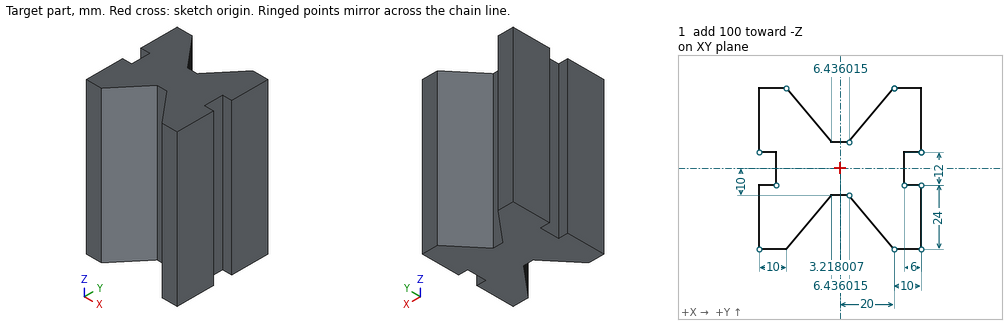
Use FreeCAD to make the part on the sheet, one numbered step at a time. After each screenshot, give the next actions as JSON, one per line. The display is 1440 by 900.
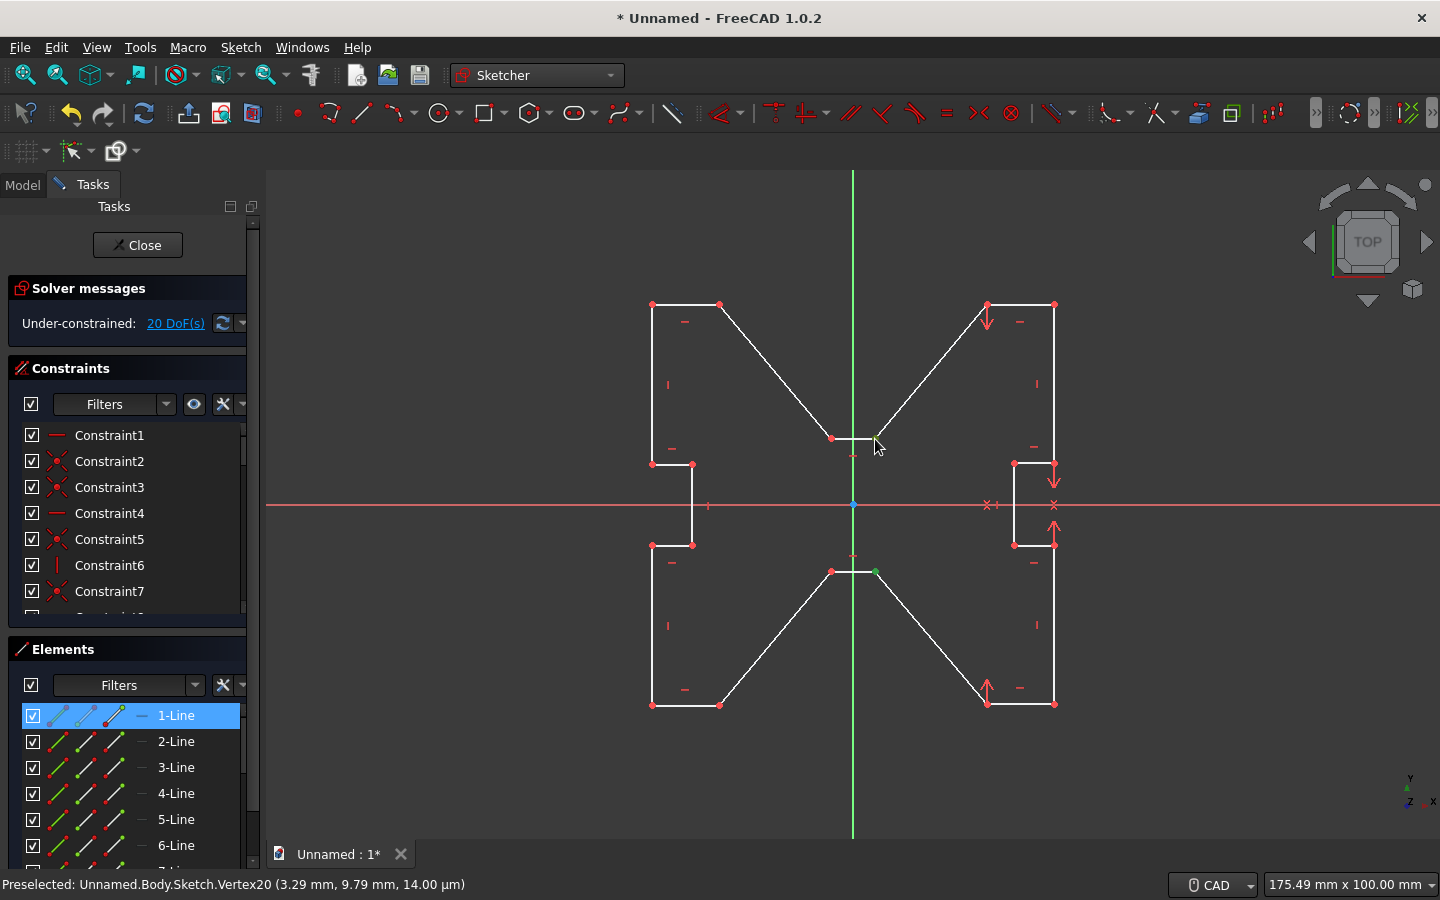
{"action": "left_click", "coordinate": [364, 504]}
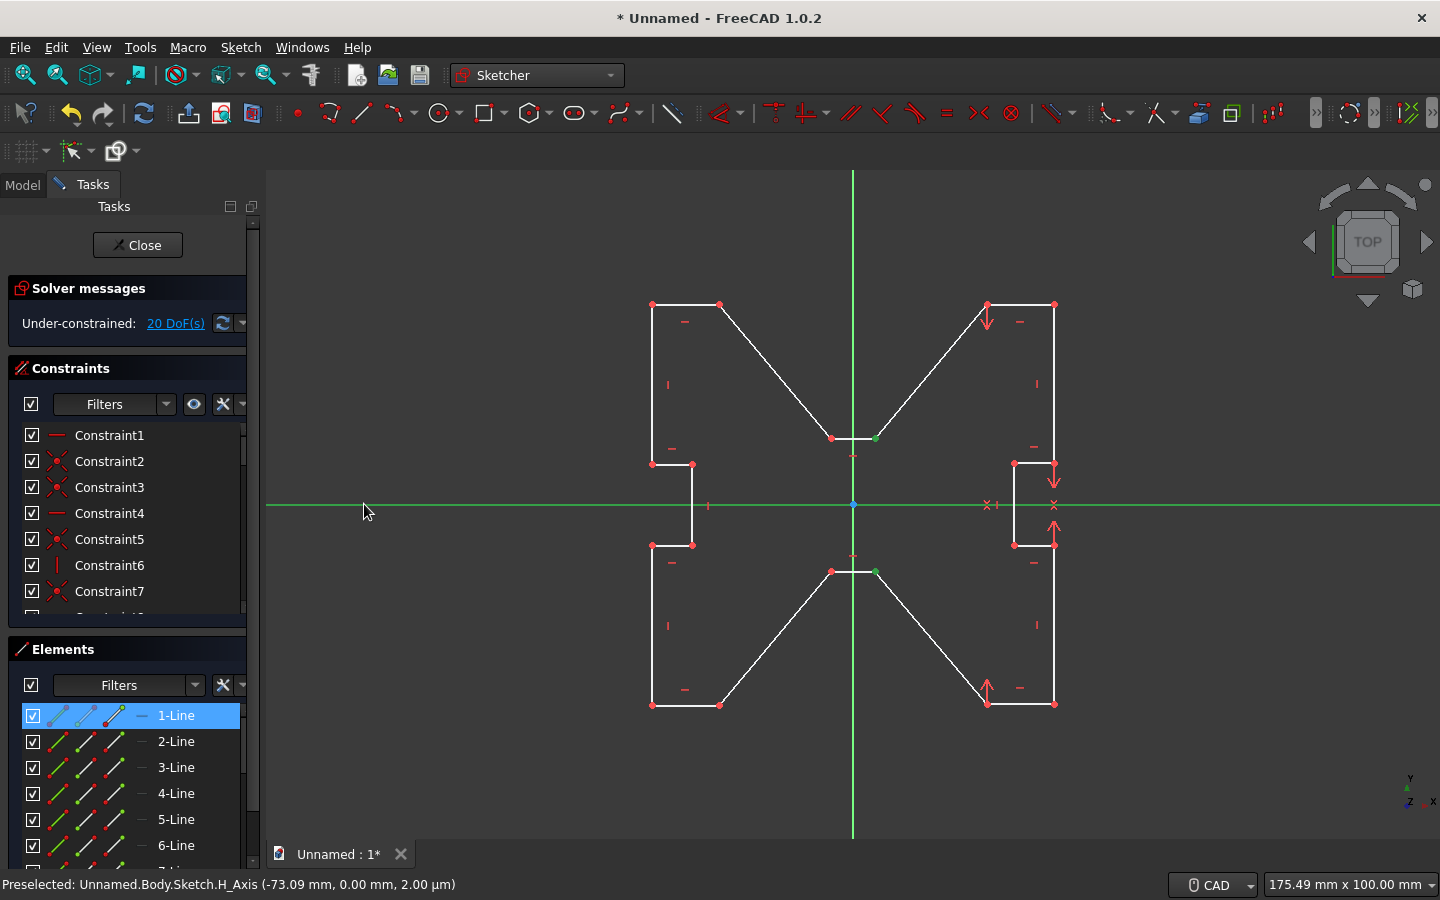
{"action": "key", "text": "s"}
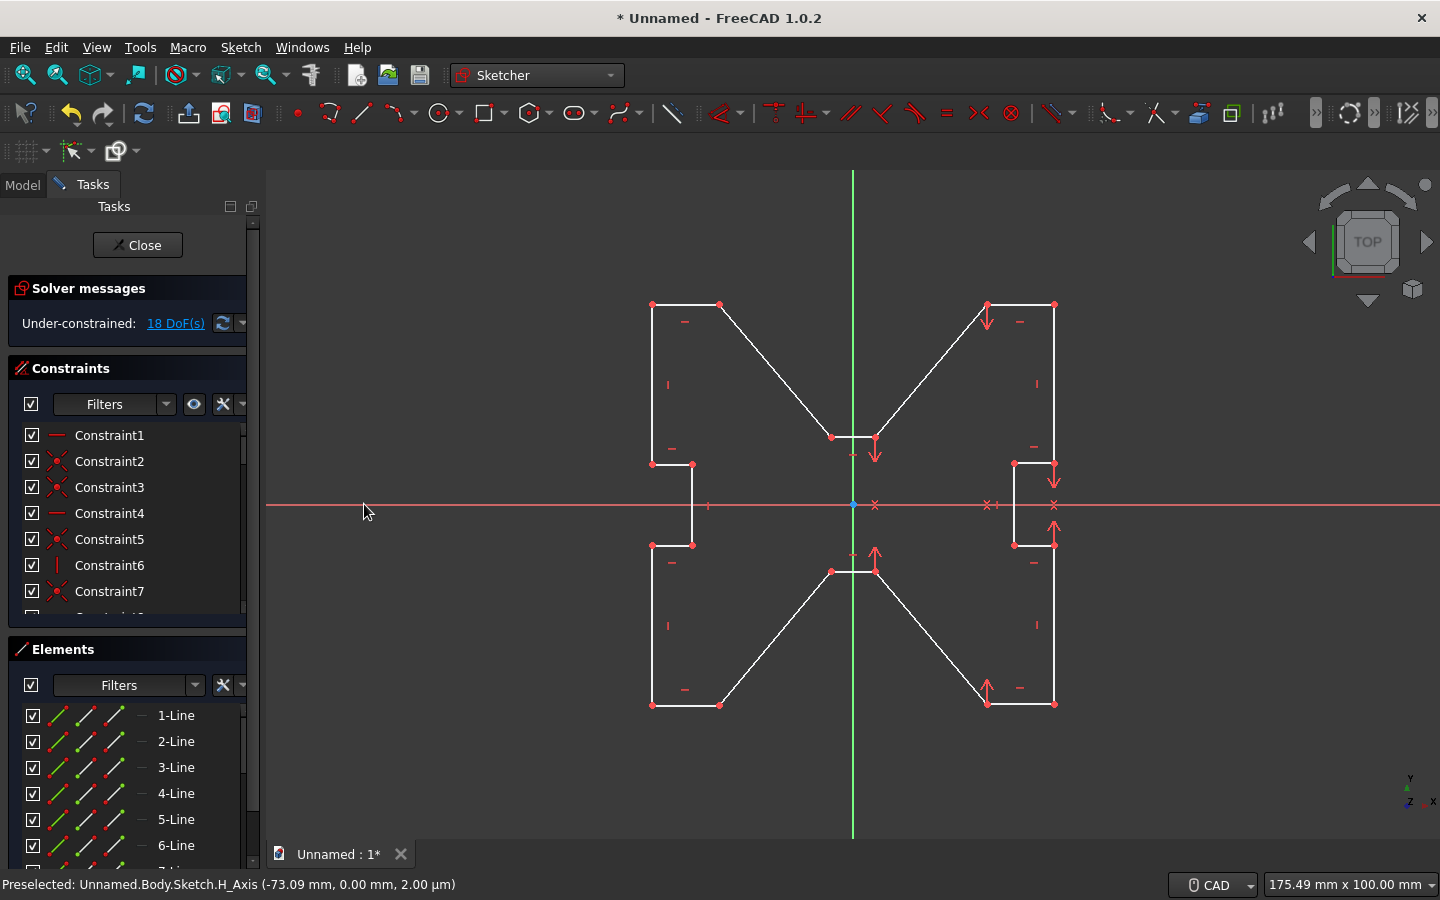
{"action": "left_click", "coordinate": [987, 305]}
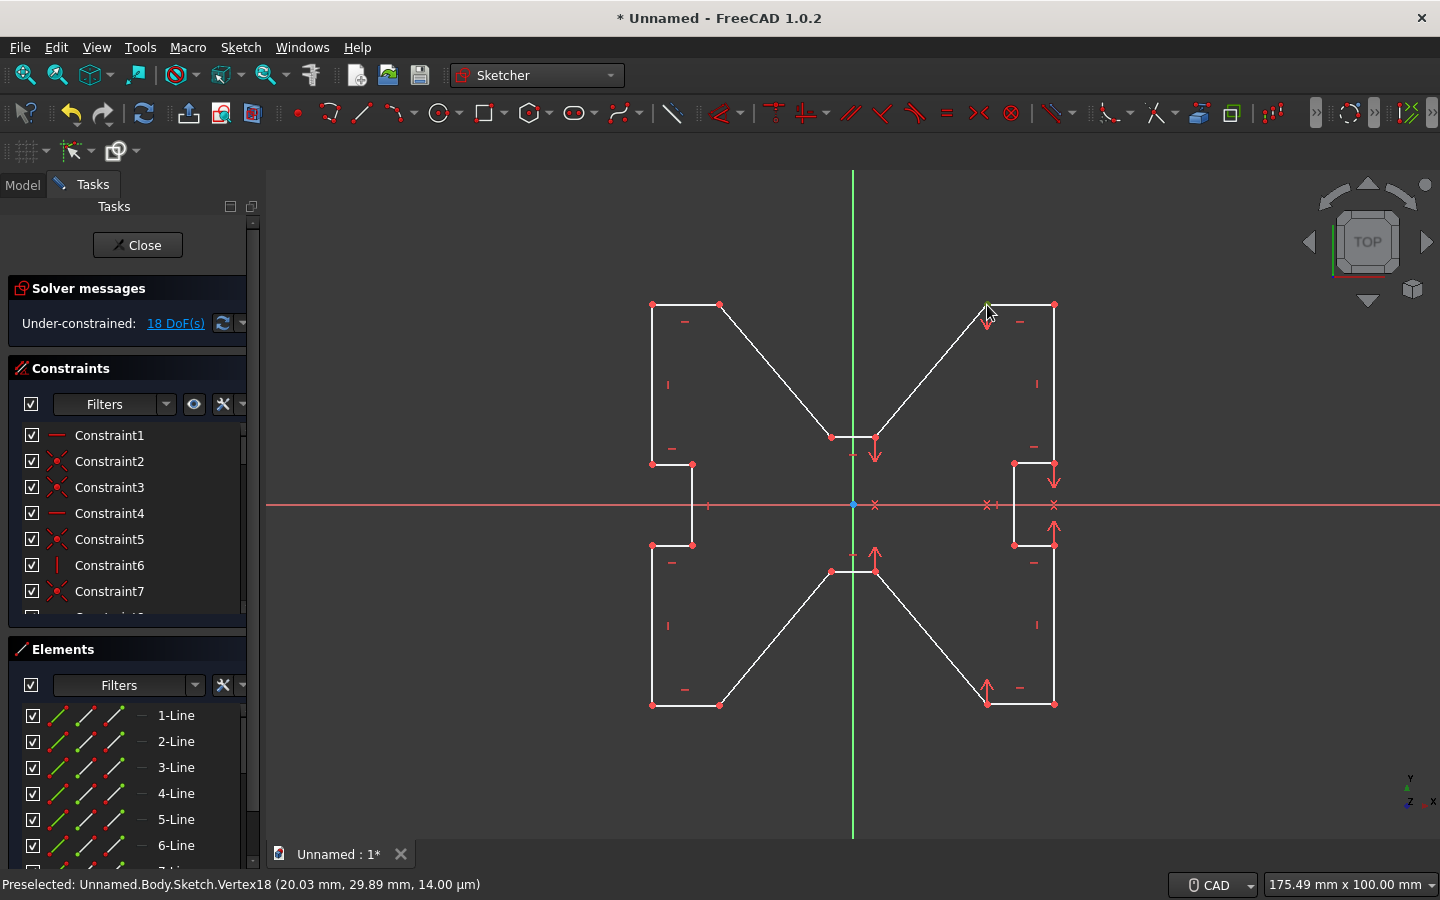
{"action": "left_click", "coordinate": [719, 305]}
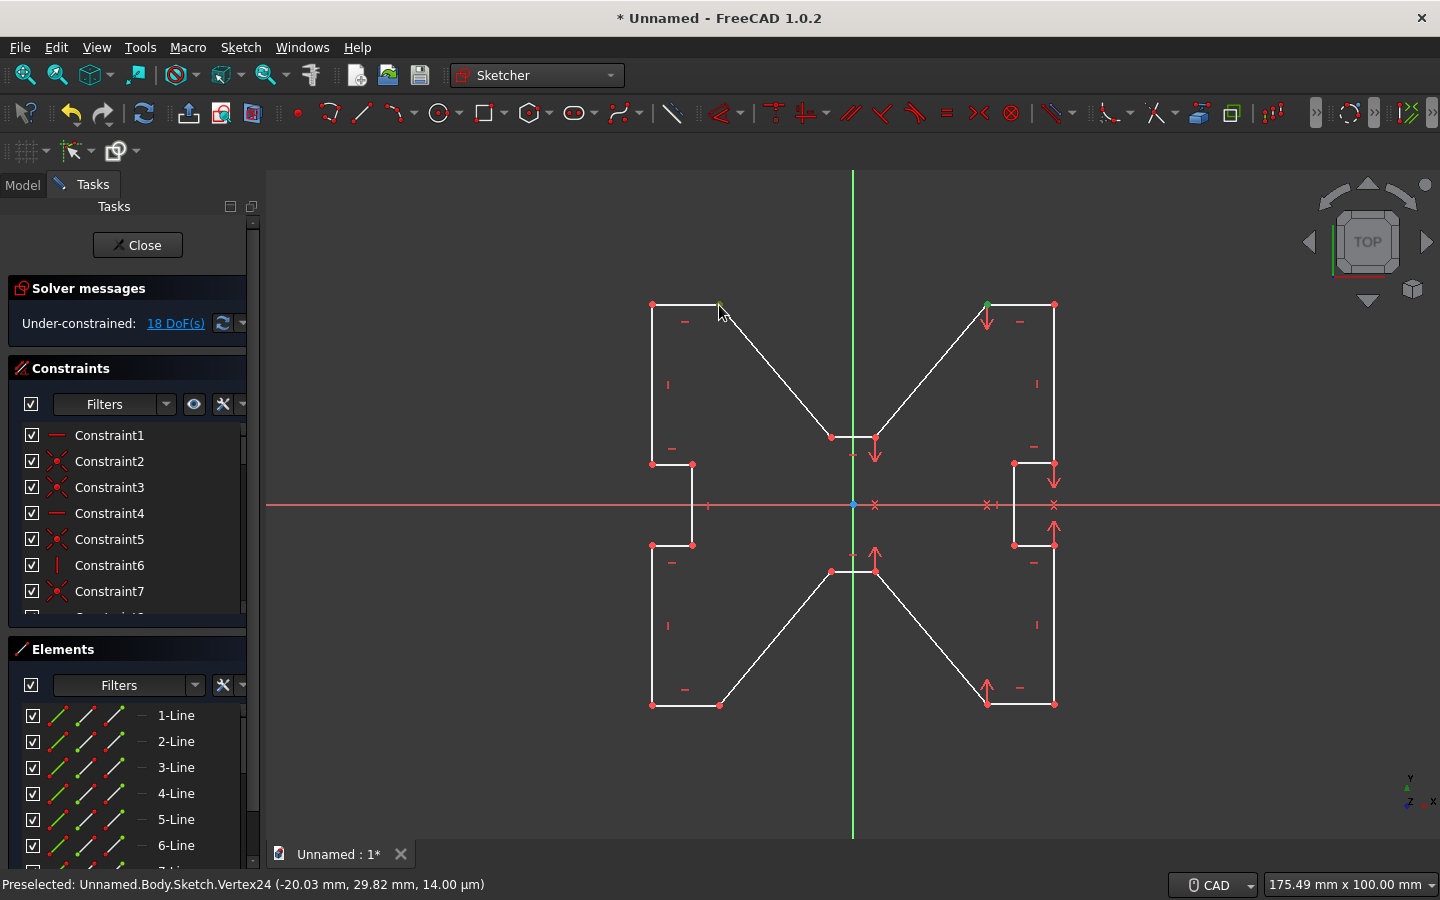
{"action": "left_click", "coordinate": [853, 767]}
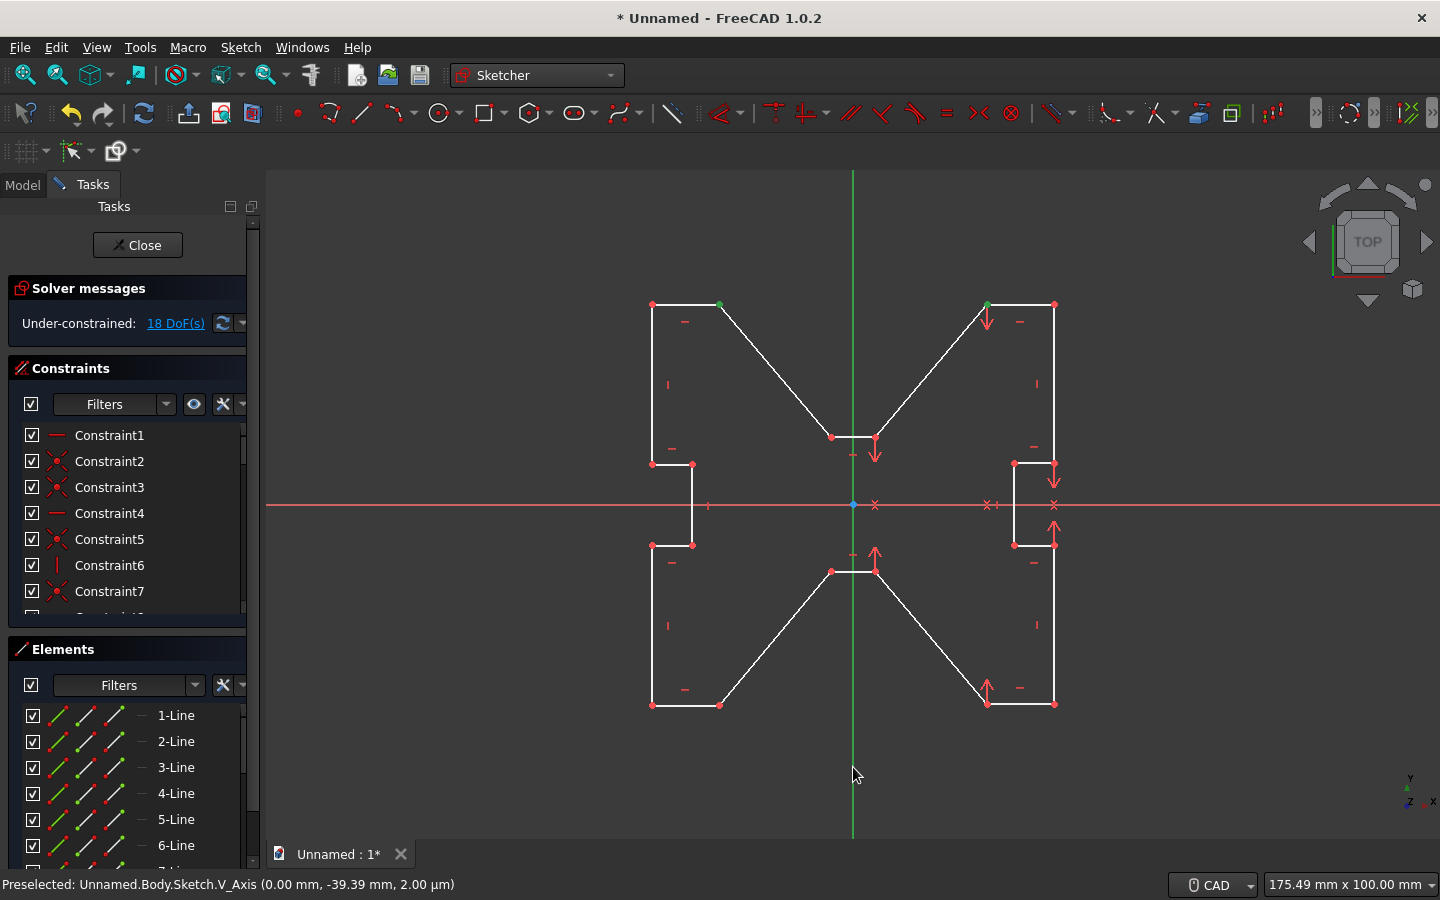
{"action": "left_click", "coordinate": [980, 114]}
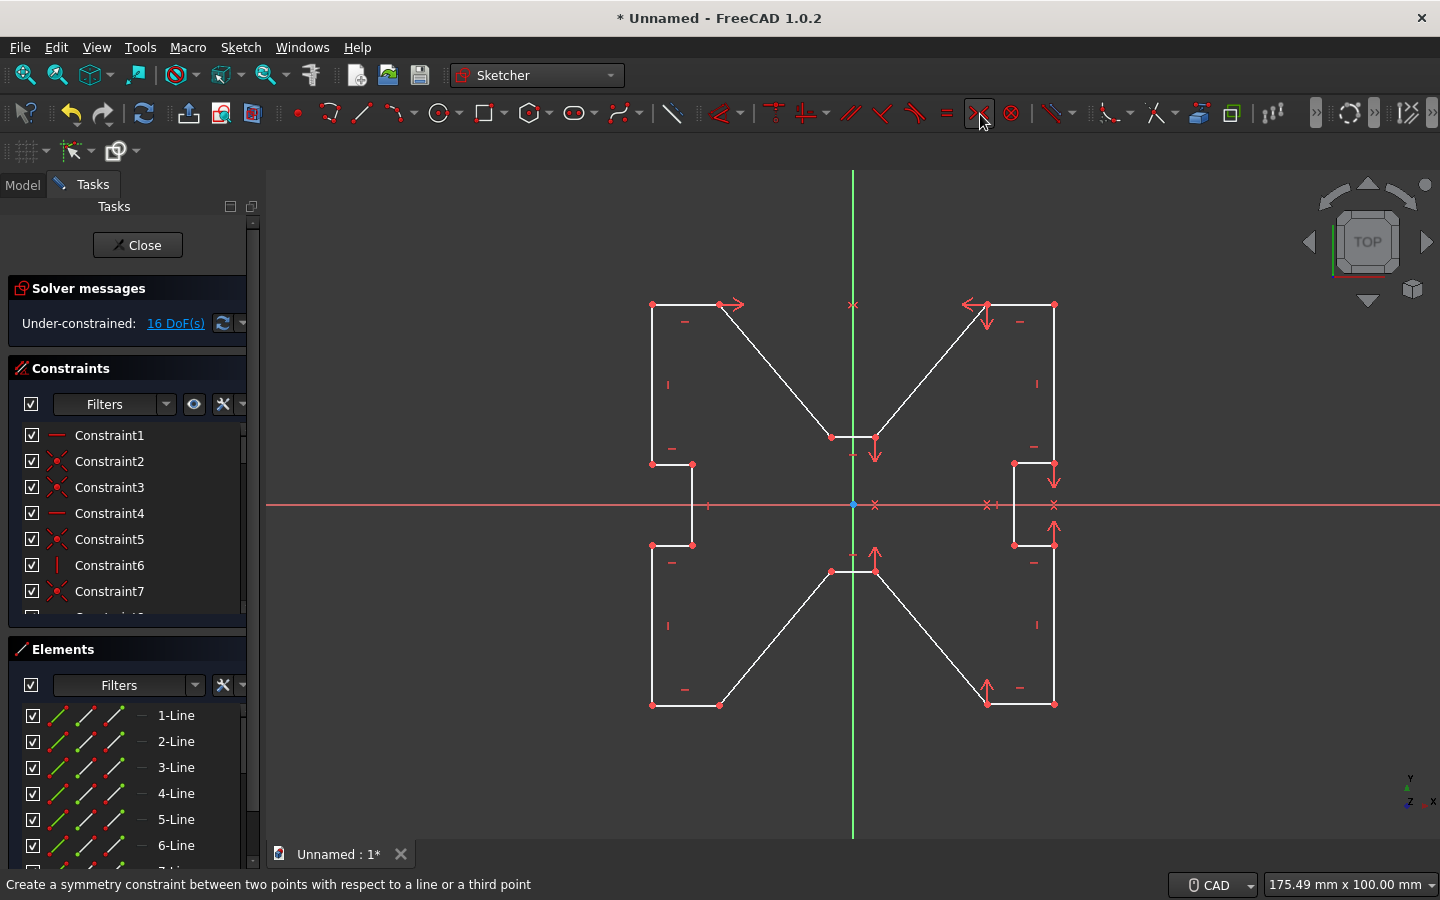
{"action": "left_click", "coordinate": [1054, 463]}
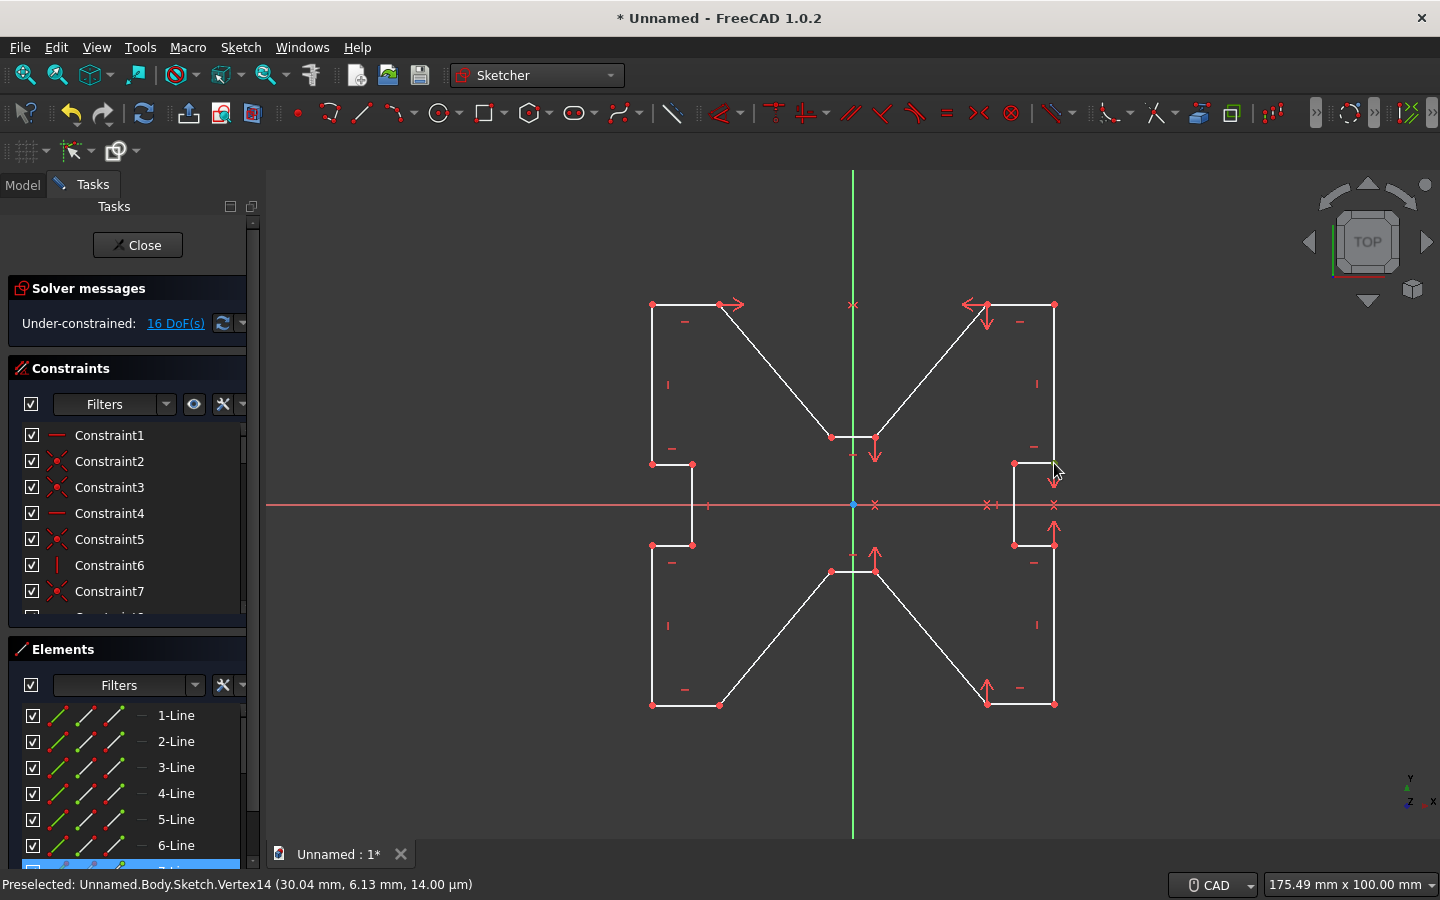
{"action": "left_click", "coordinate": [652, 465]}